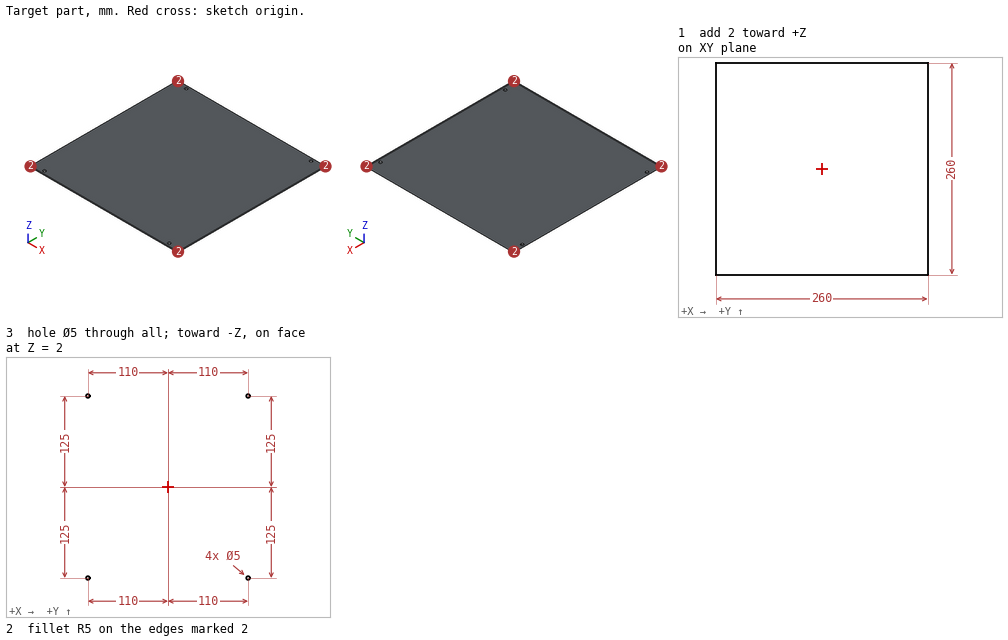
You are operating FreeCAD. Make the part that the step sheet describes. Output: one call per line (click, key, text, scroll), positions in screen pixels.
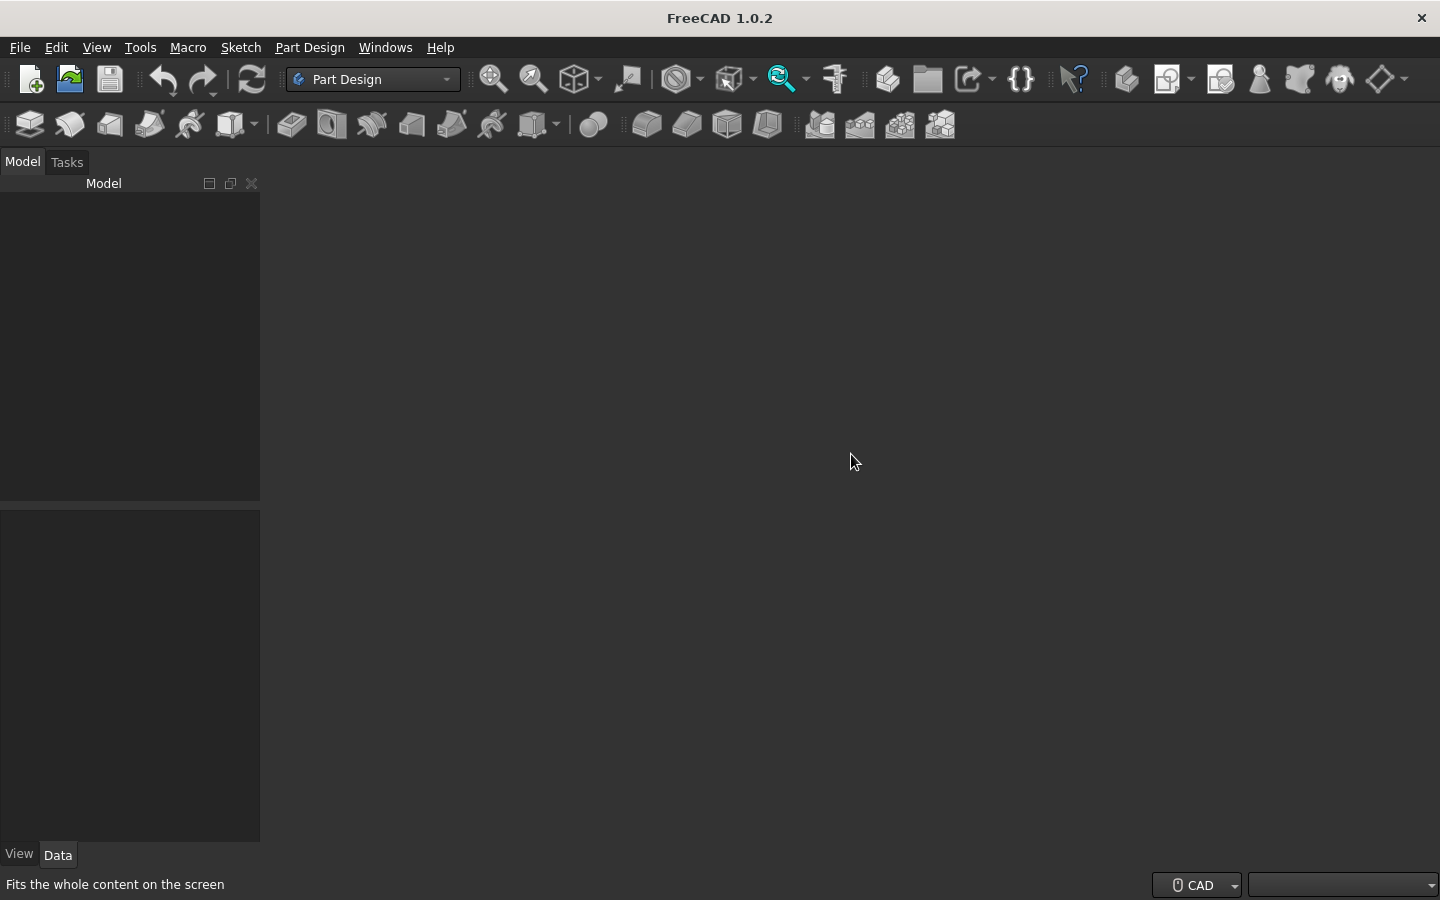
click(30, 80)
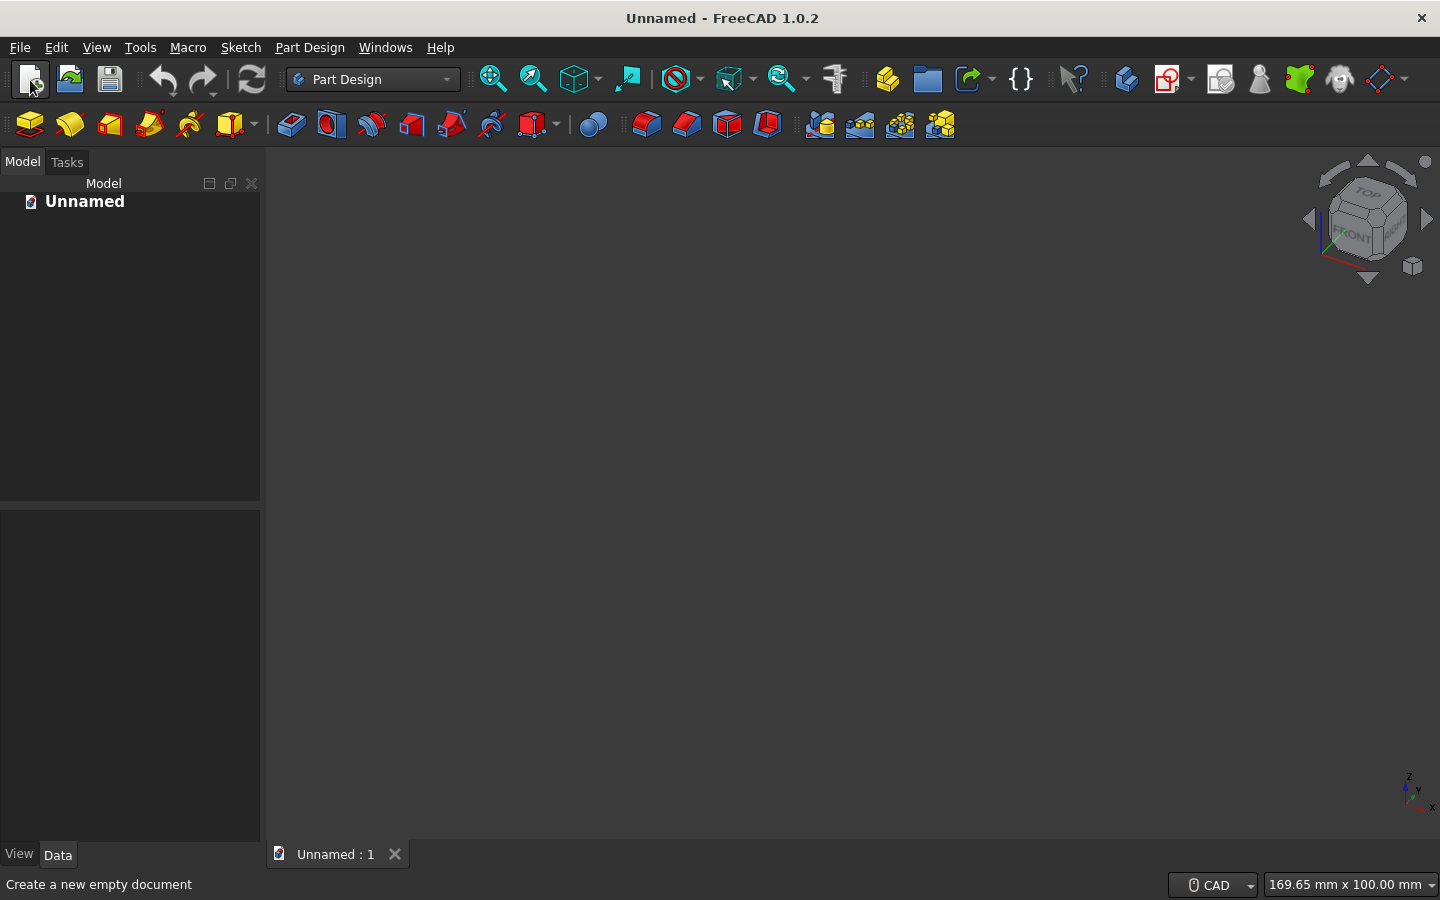
click(1168, 80)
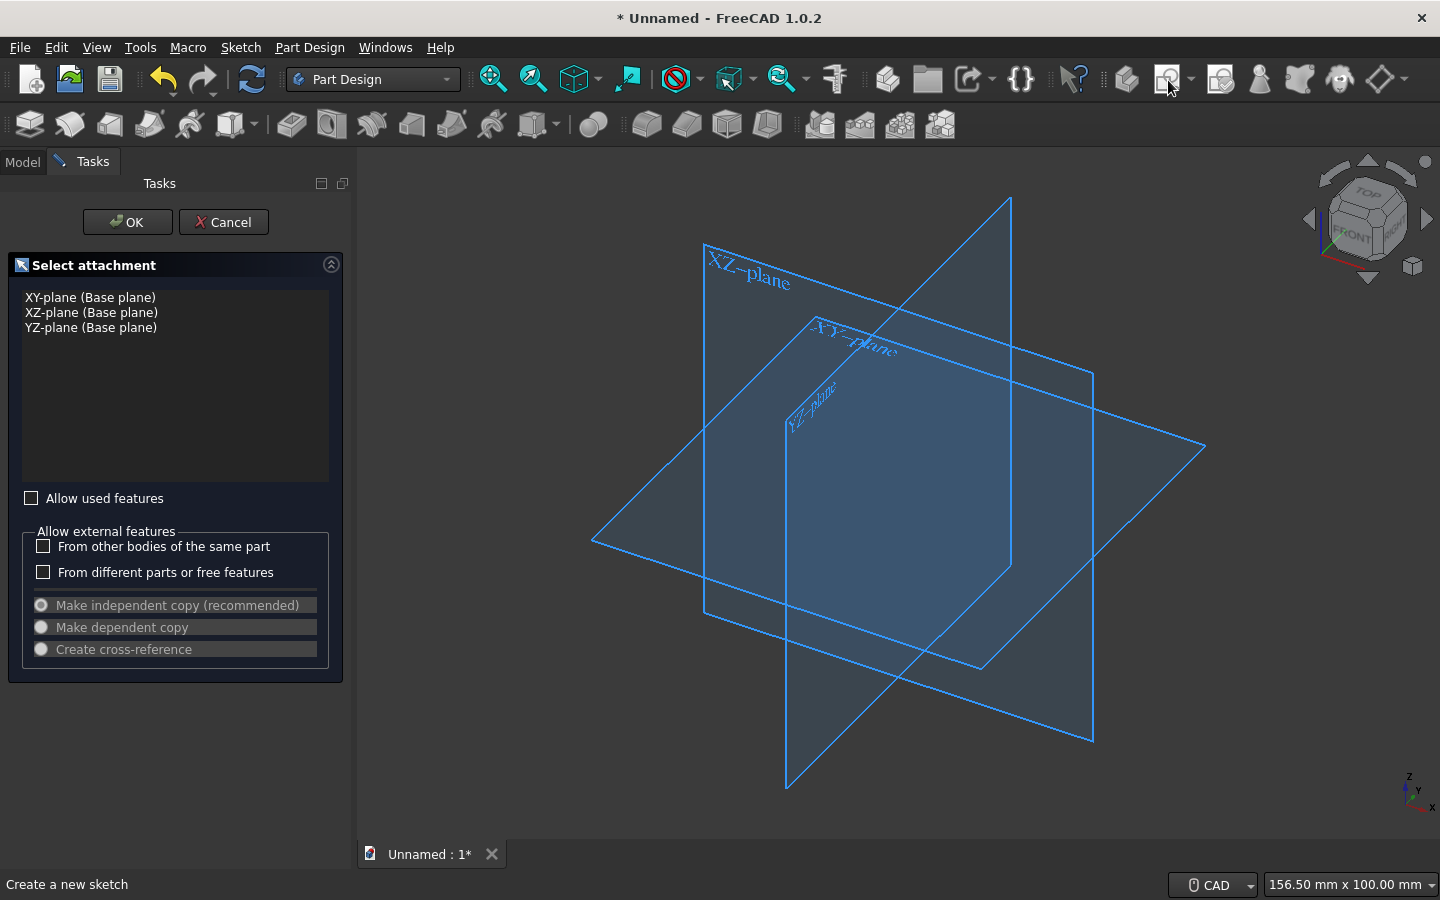
click(82, 298)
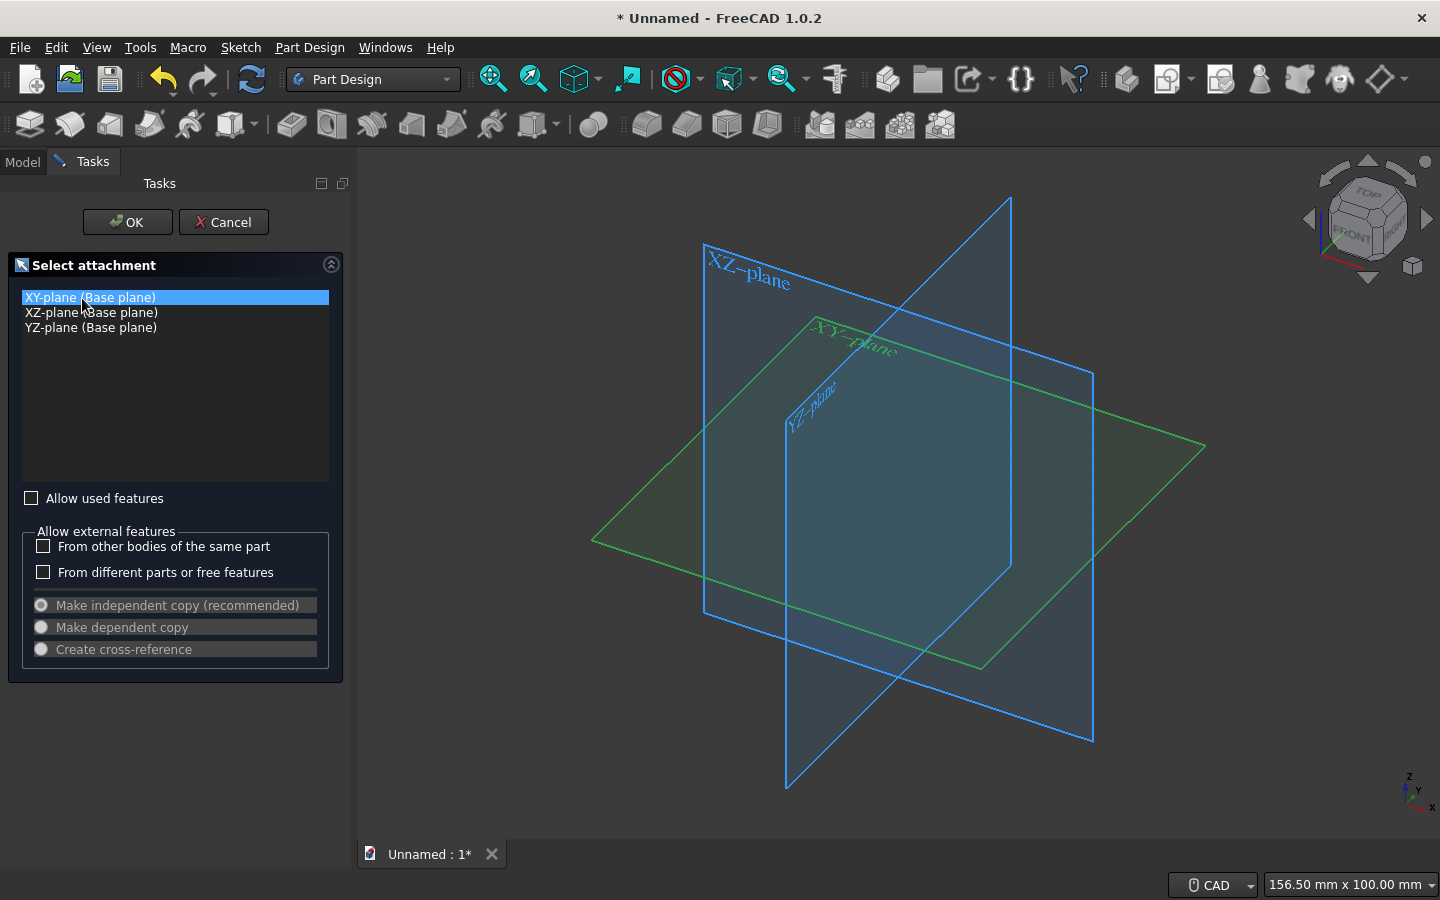
click(128, 222)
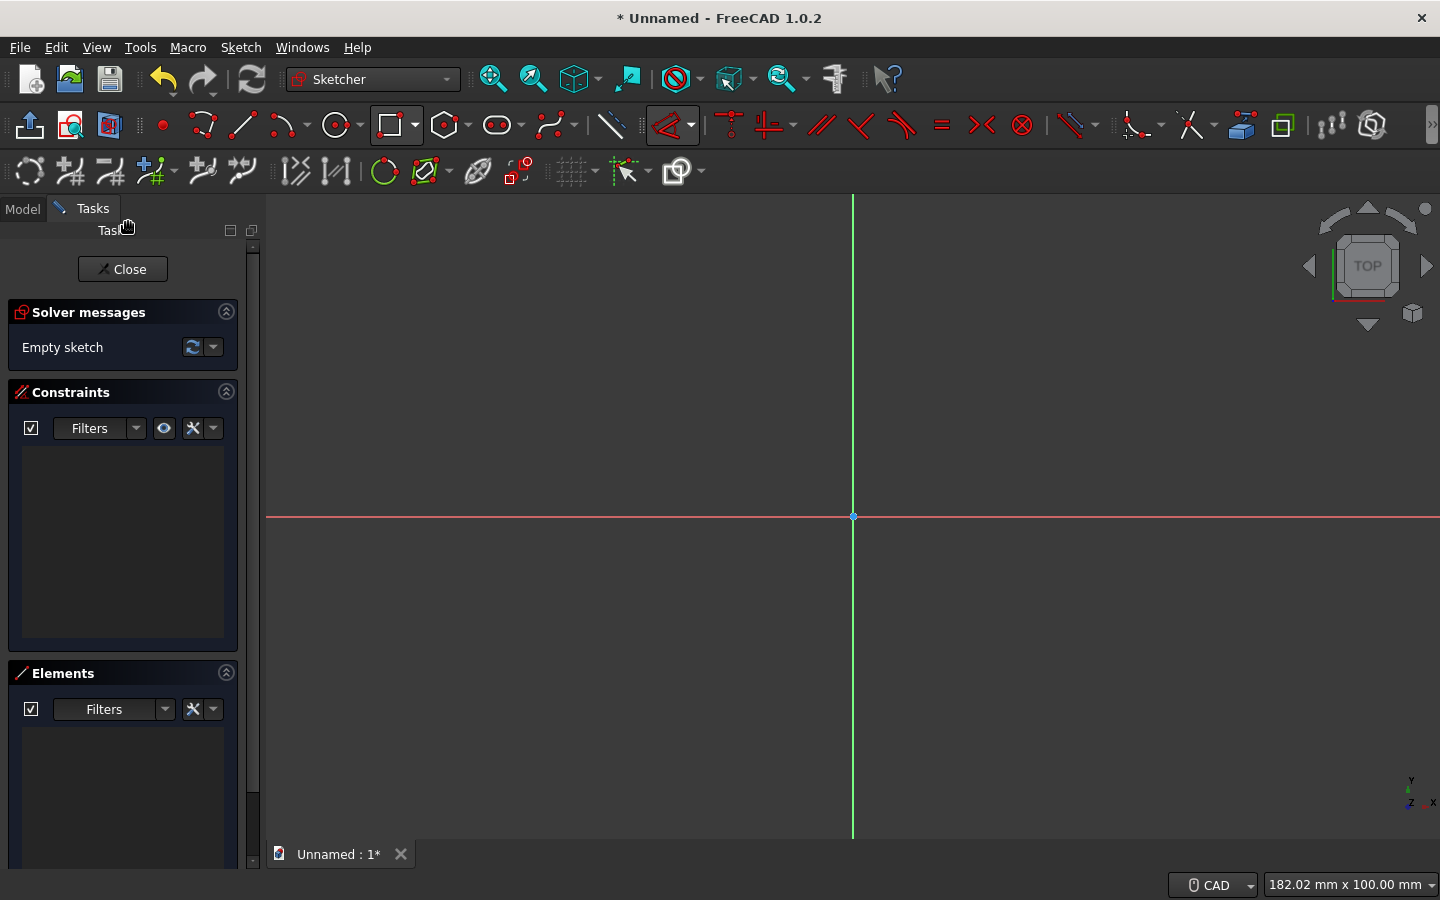
scroll(762, 516, down, 7)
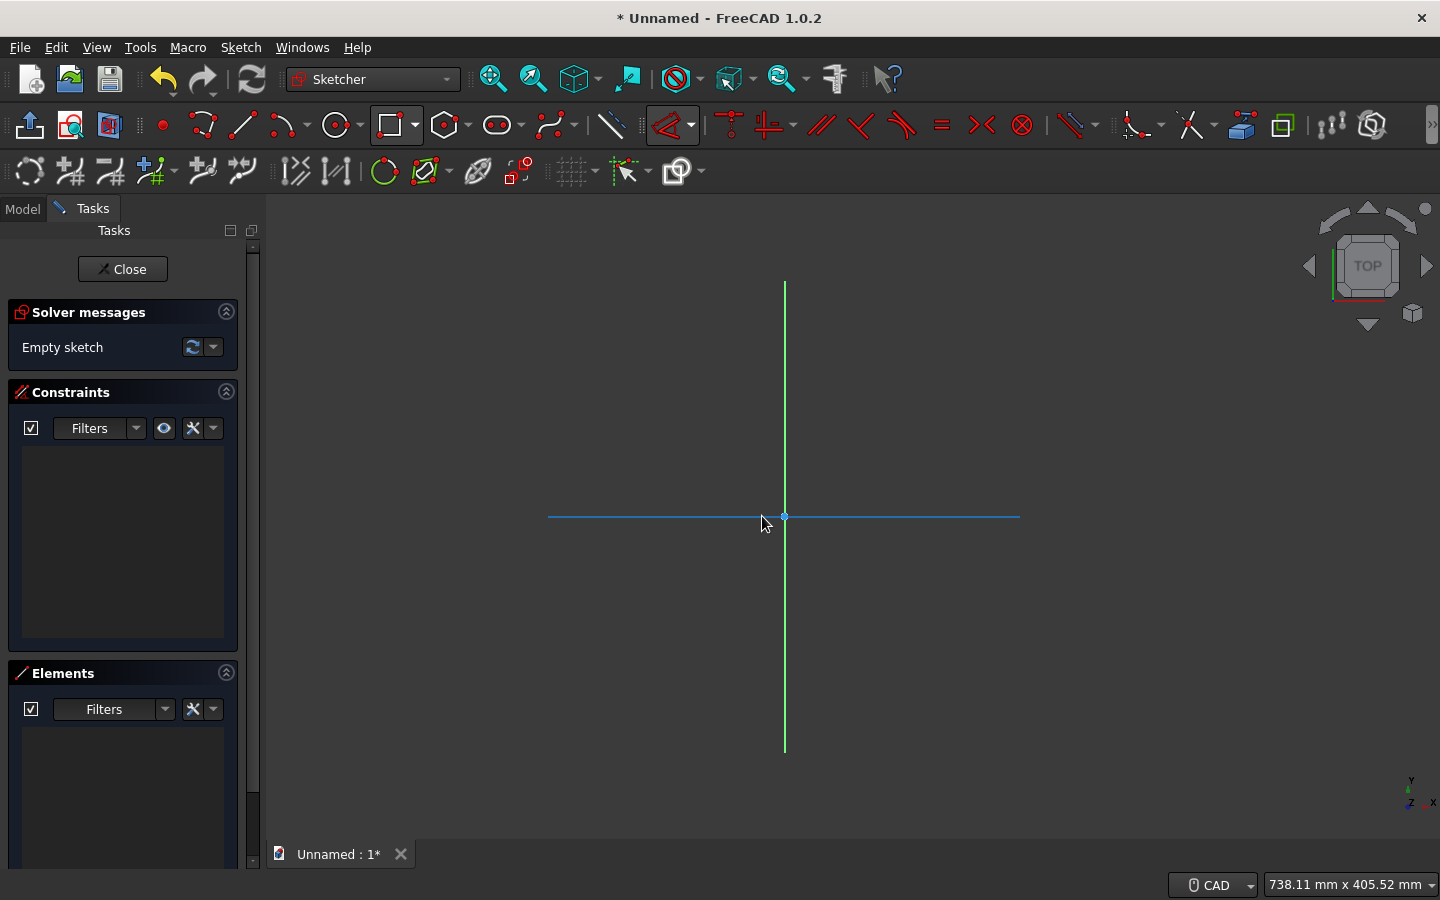
click(418, 126)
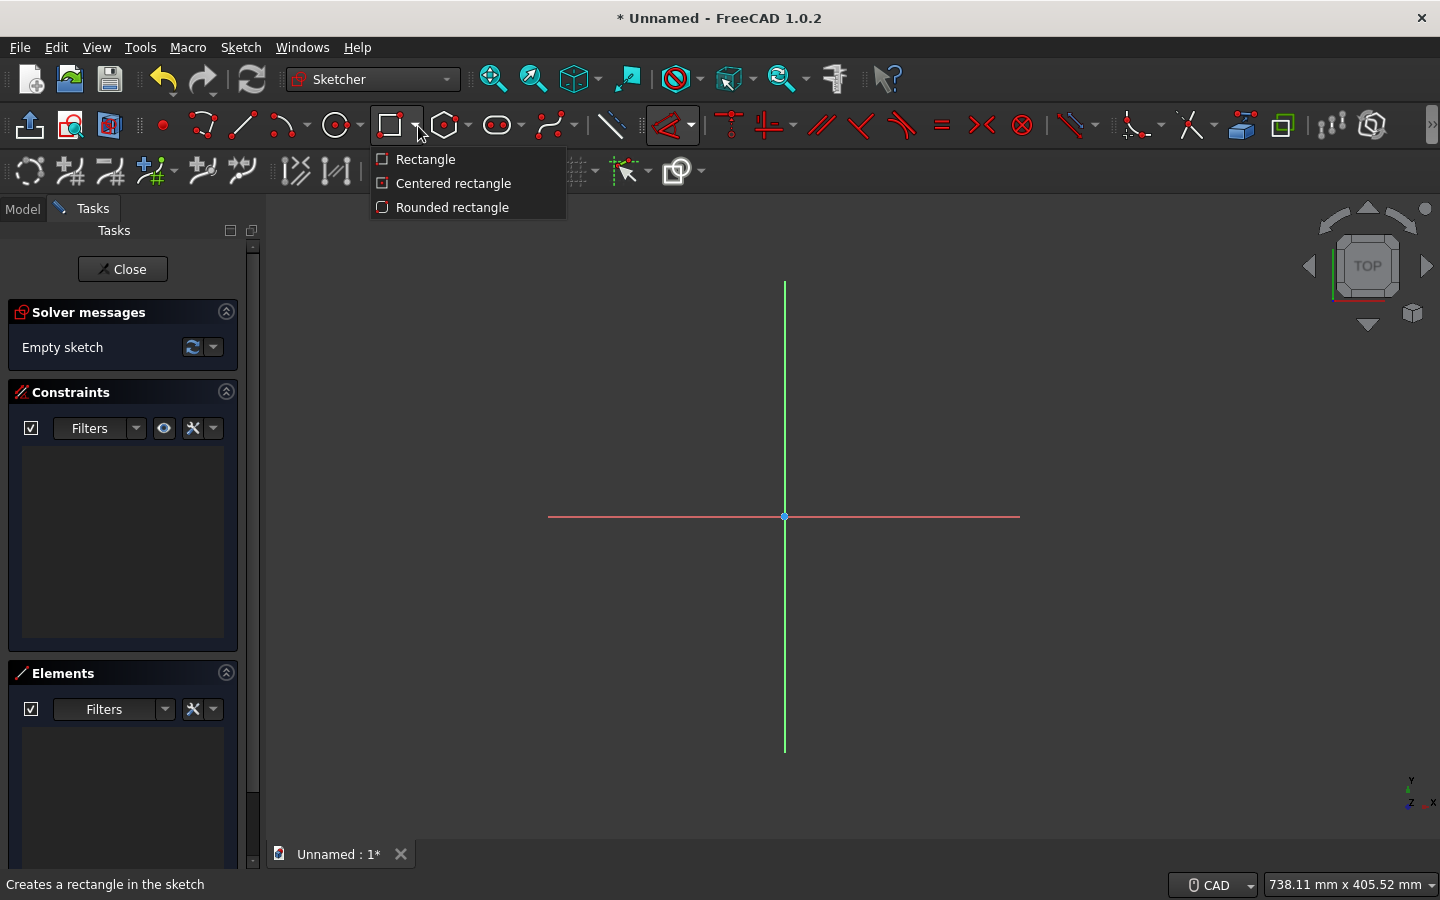
click(468, 183)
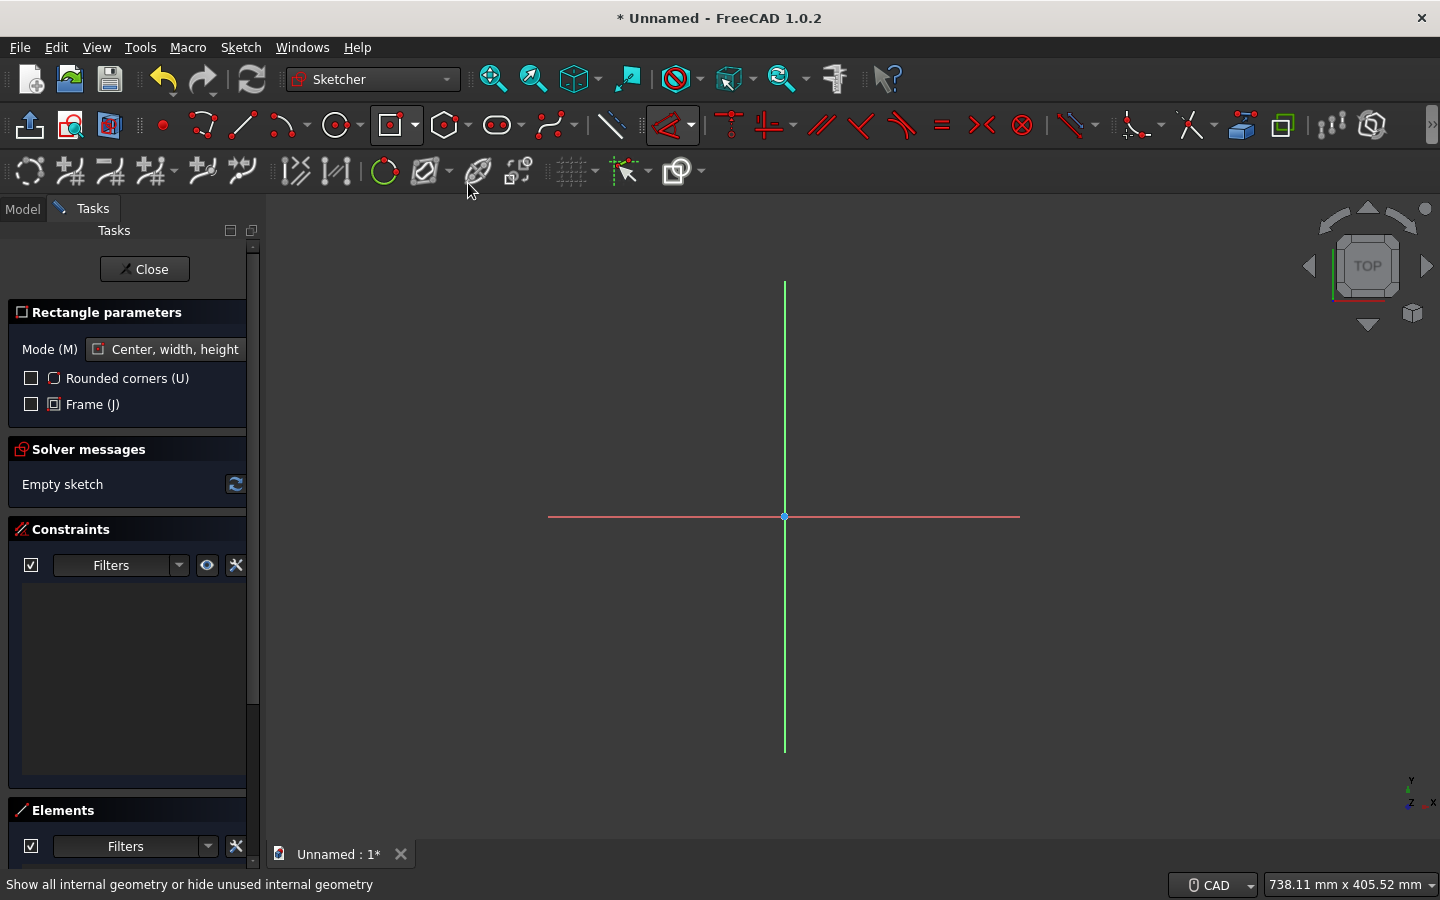
click(785, 516)
move(992, 310)